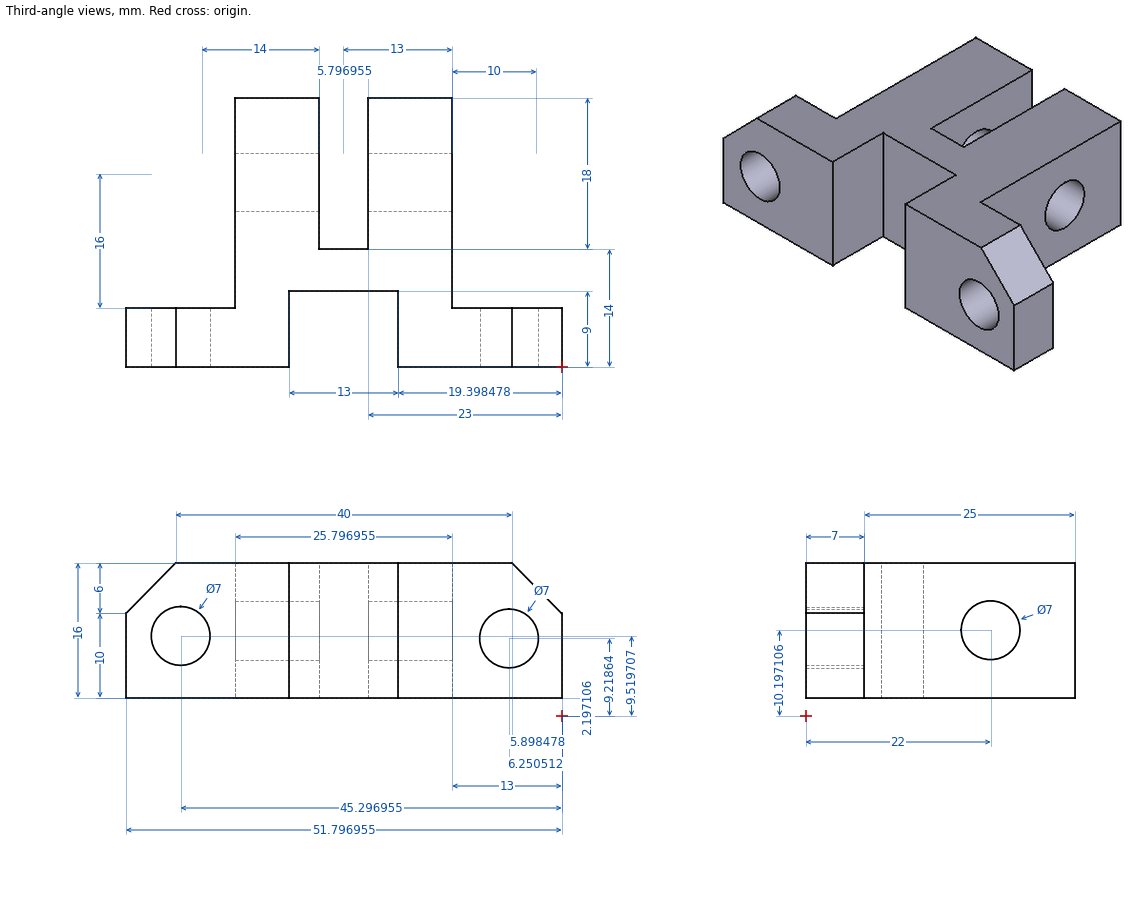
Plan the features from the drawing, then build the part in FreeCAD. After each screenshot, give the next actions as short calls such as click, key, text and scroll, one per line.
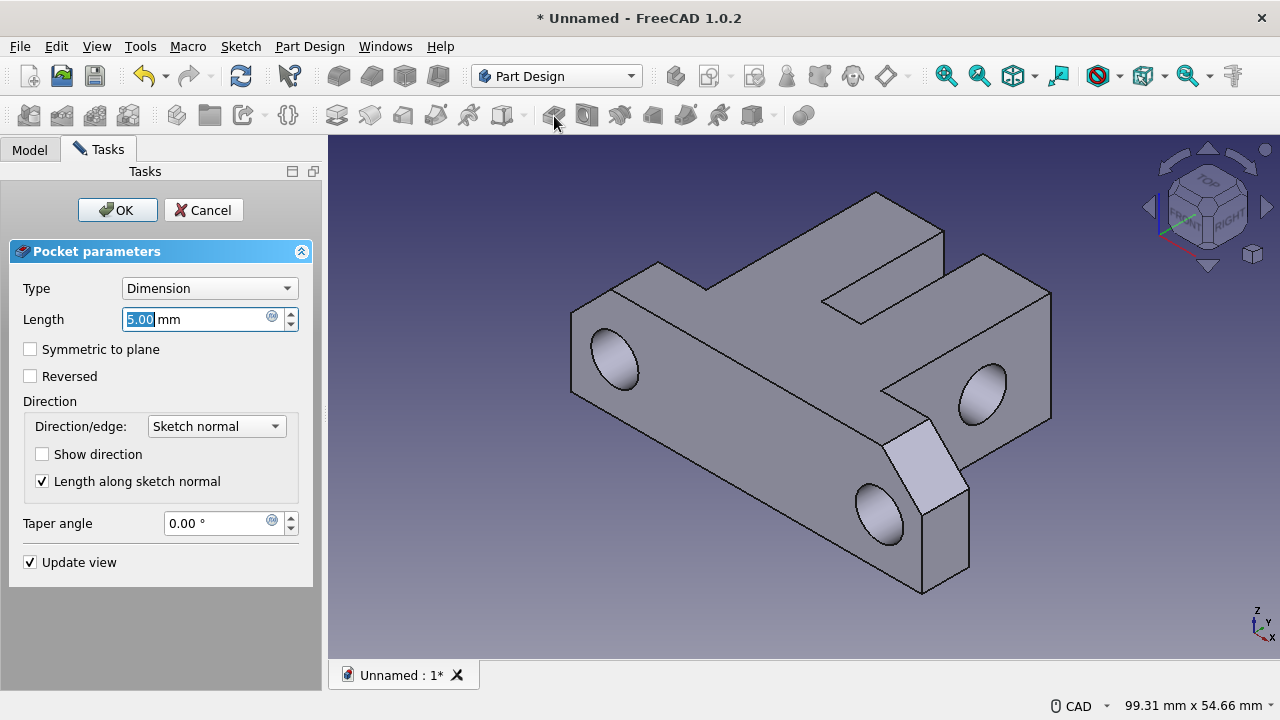
click(210, 288)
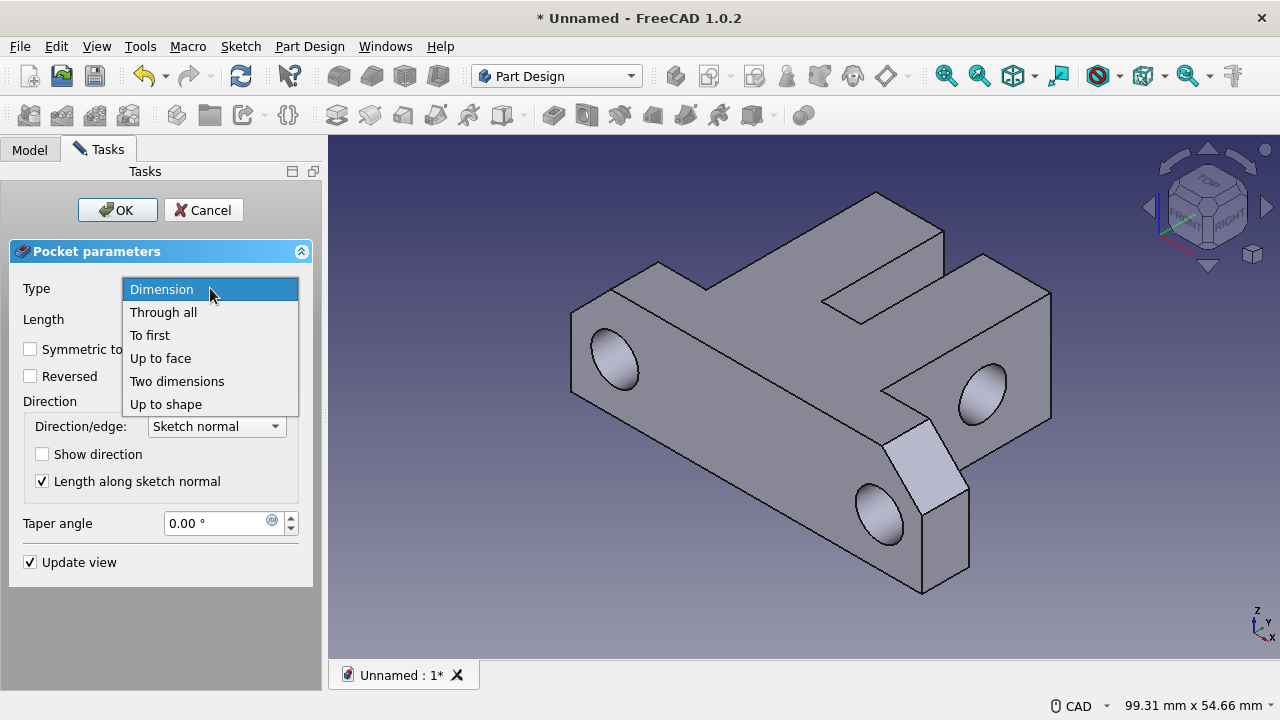
click(208, 382)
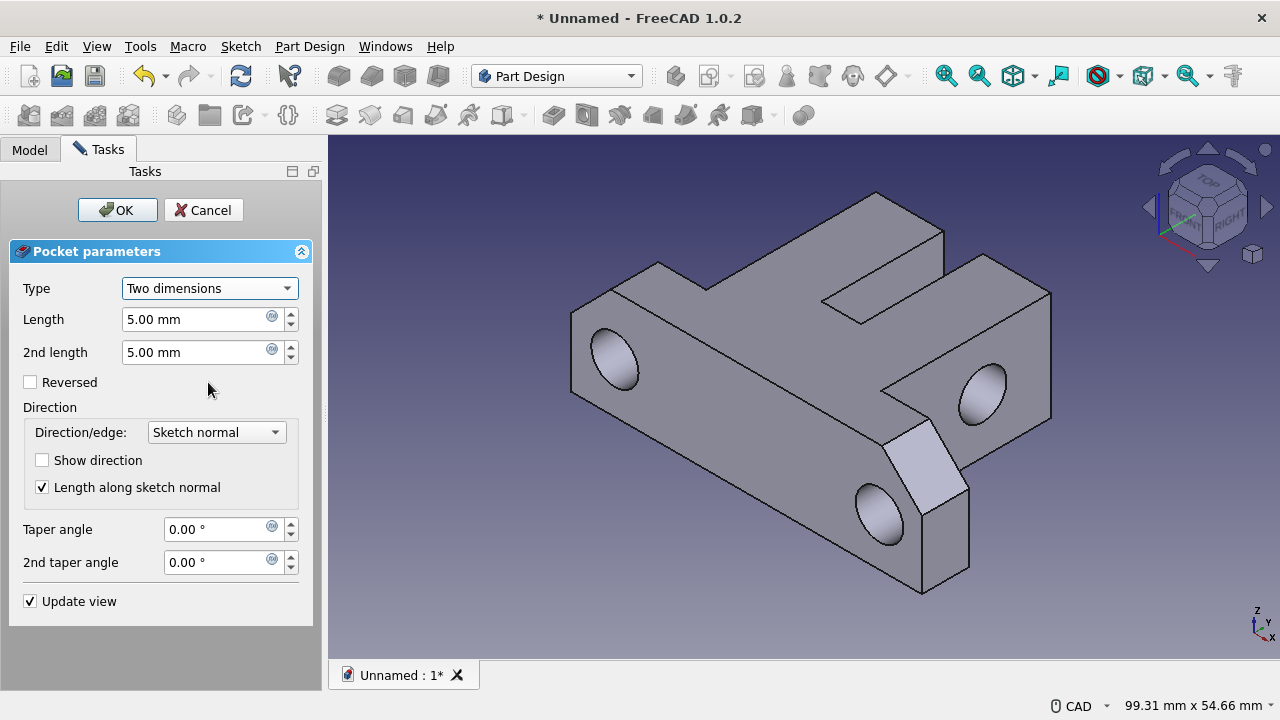
triple_click(204, 320)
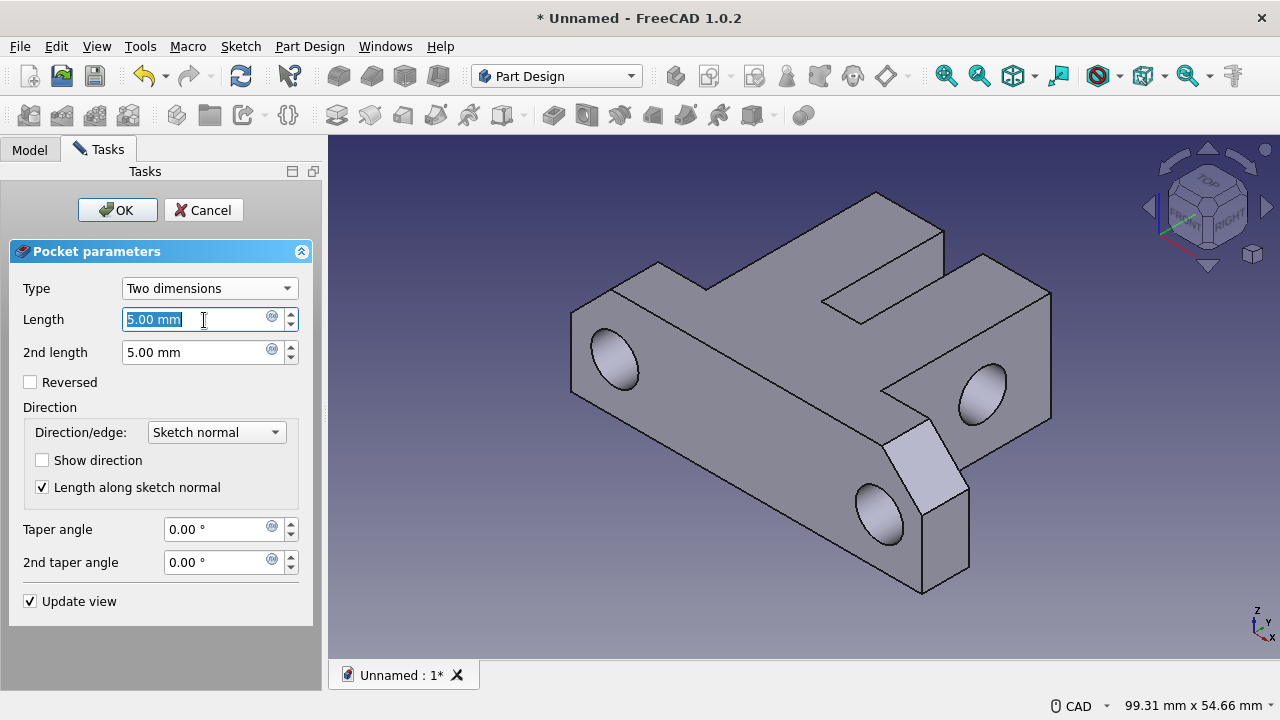
text(10)
key(Tab)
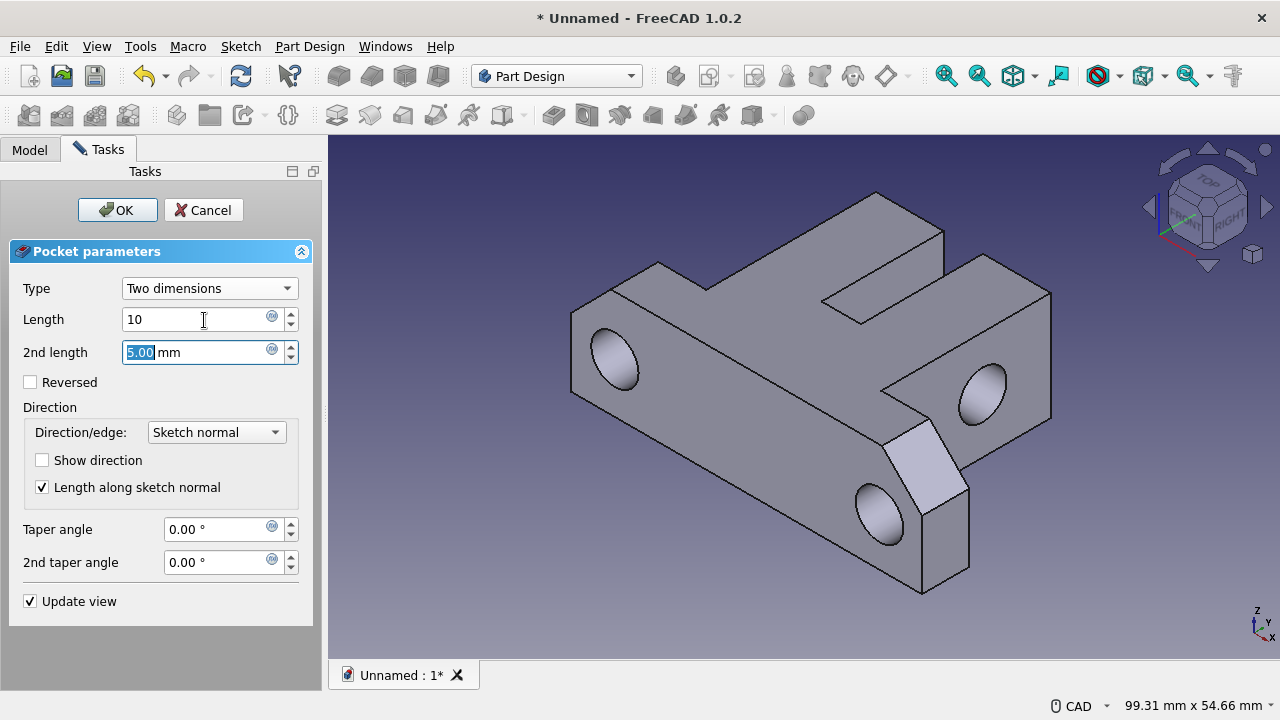
text(13)
key(Tab)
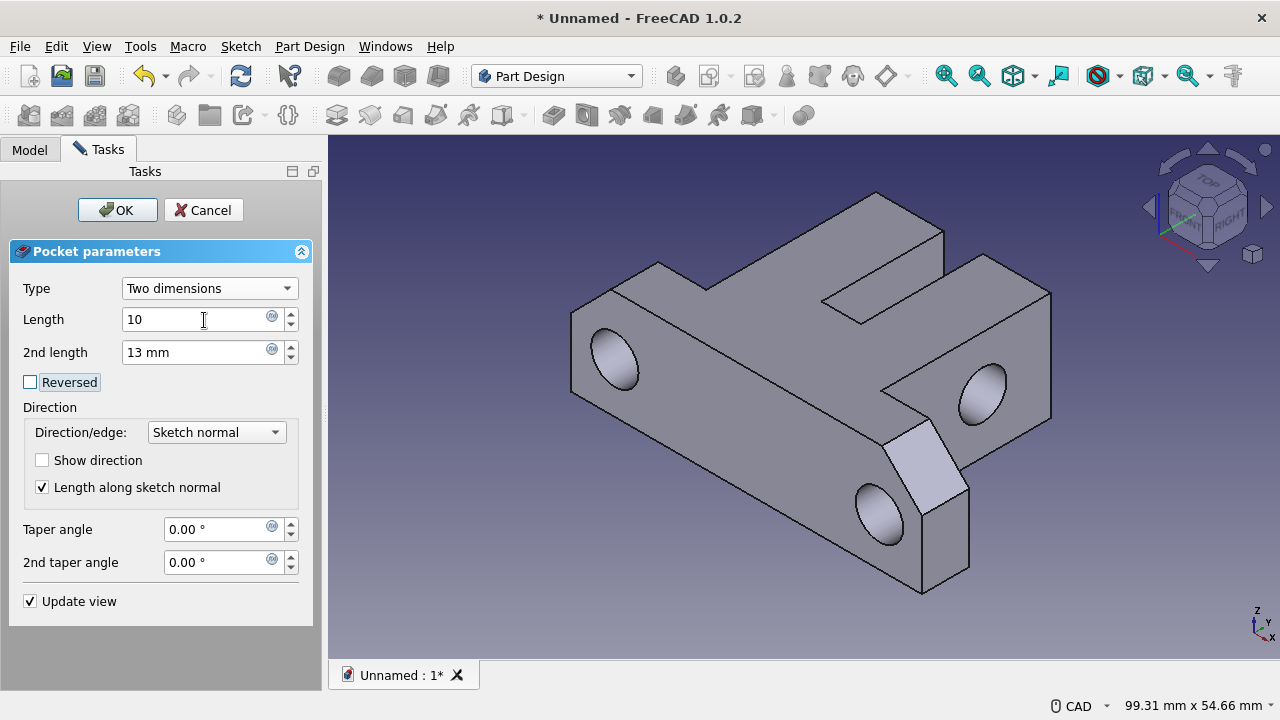
click(31, 382)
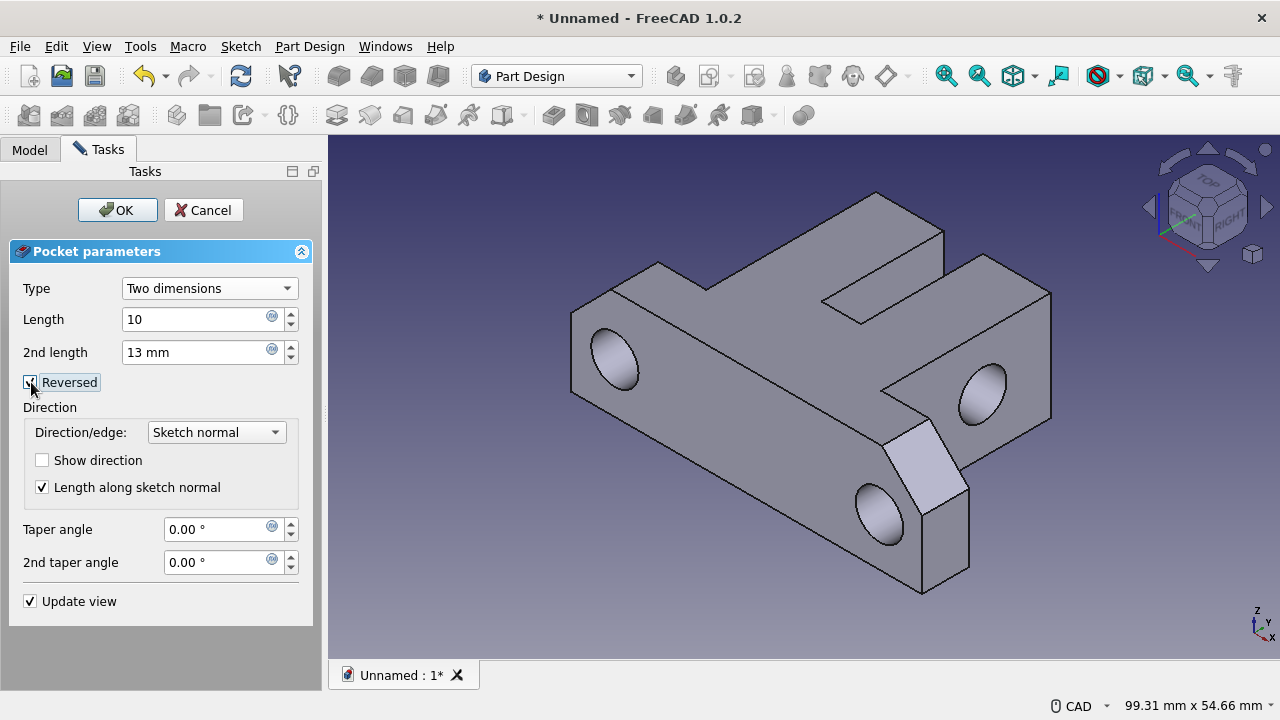
click(118, 210)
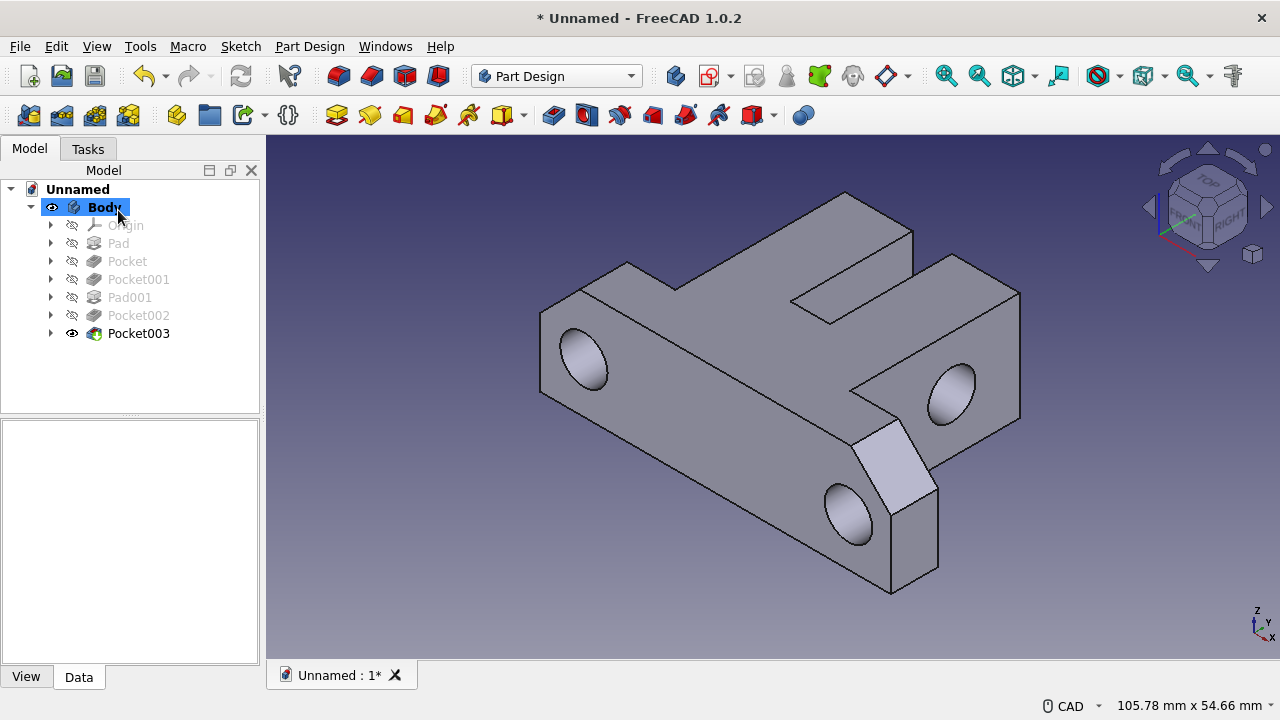
key(3)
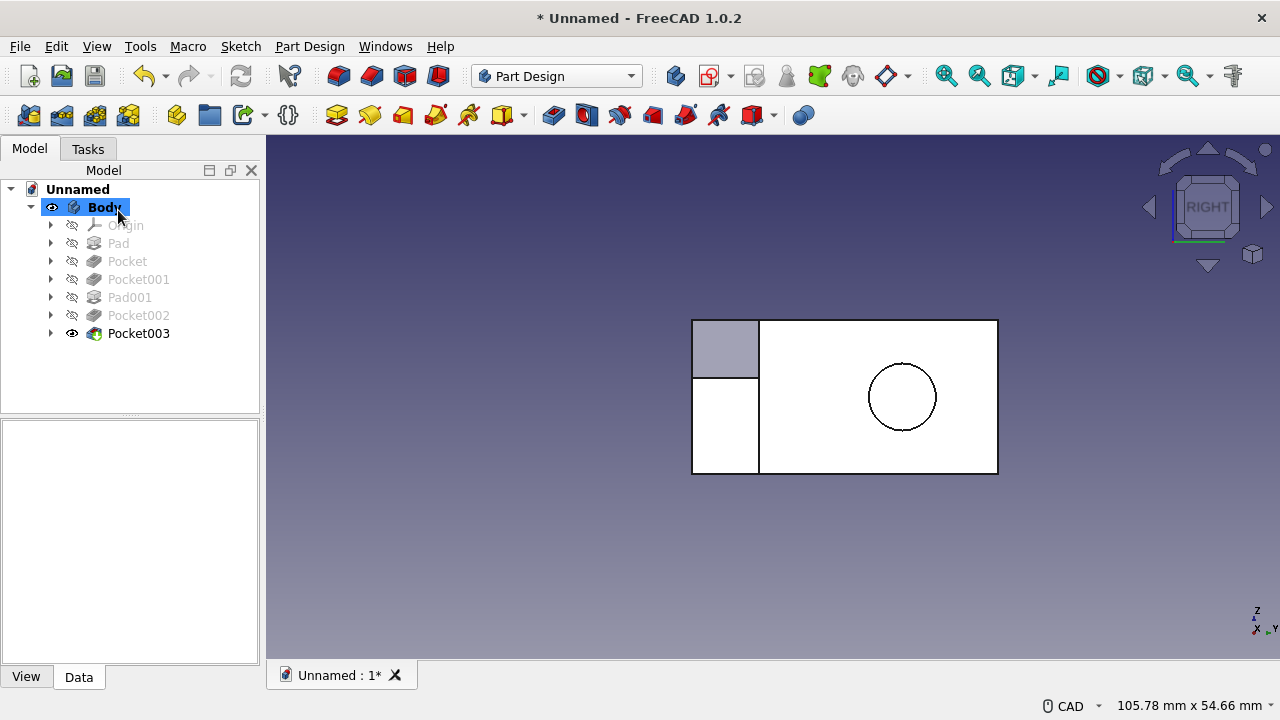
click(947, 76)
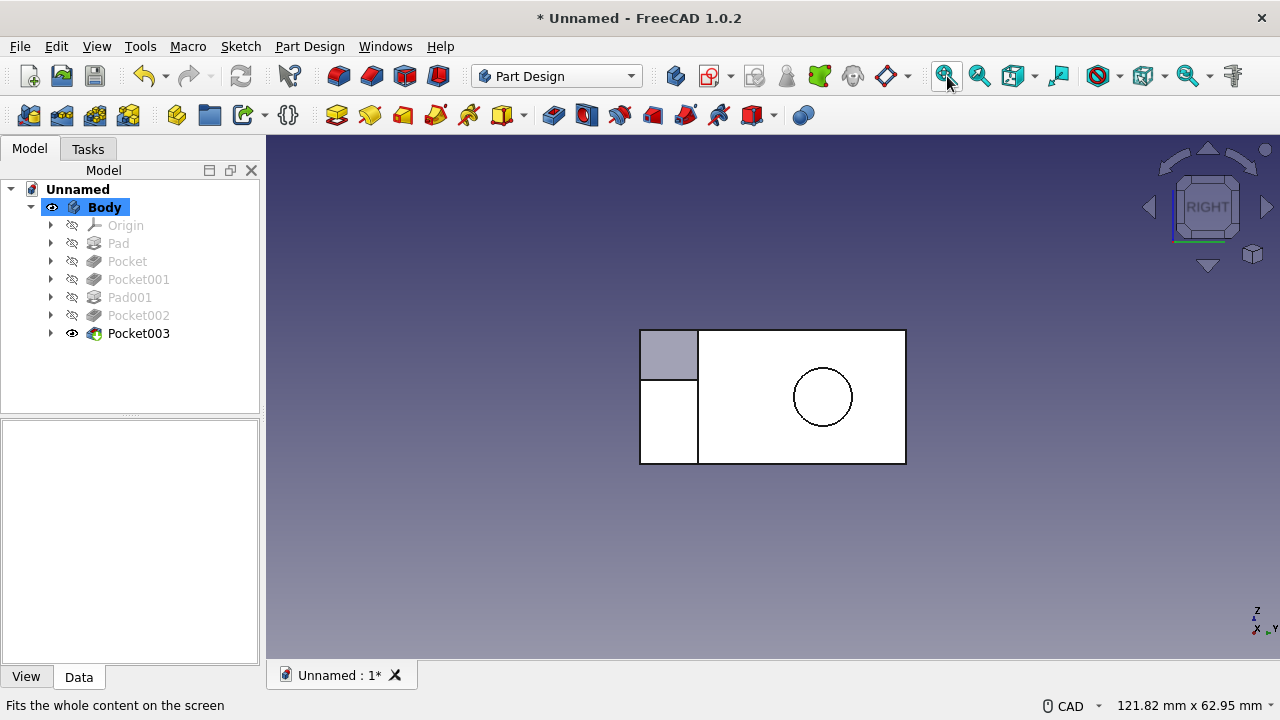
click(831, 396)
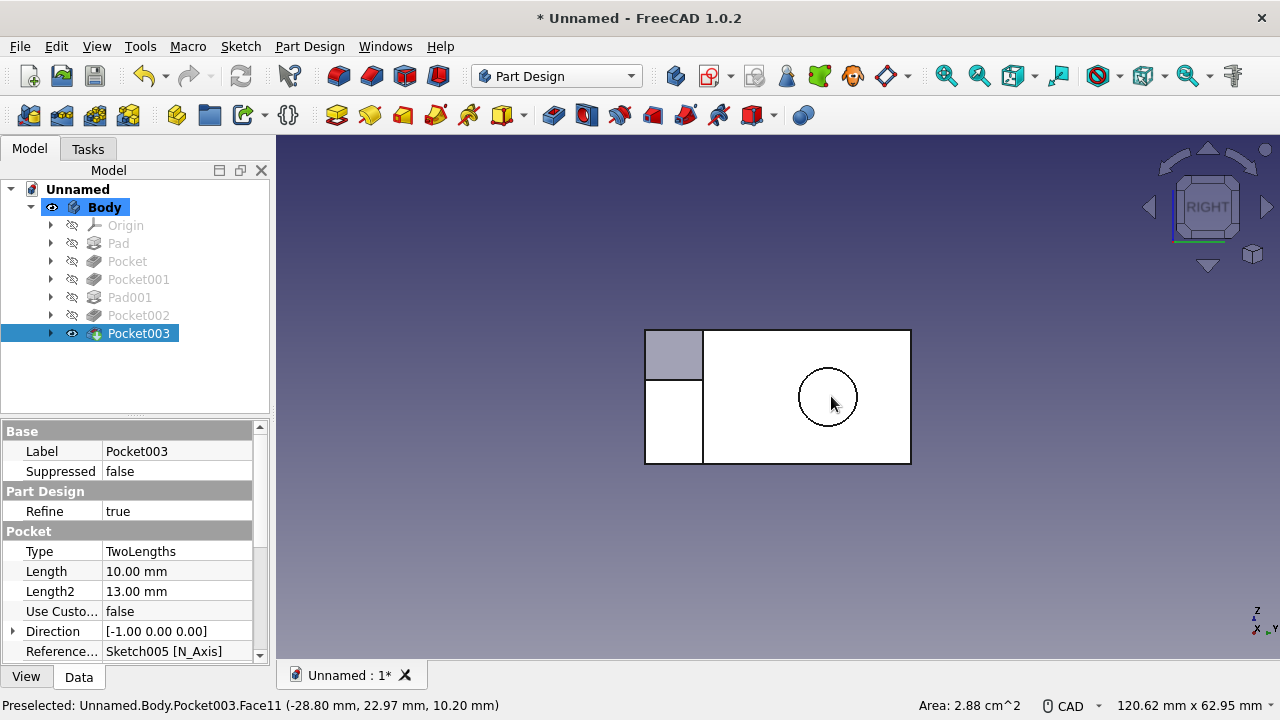
click(708, 76)